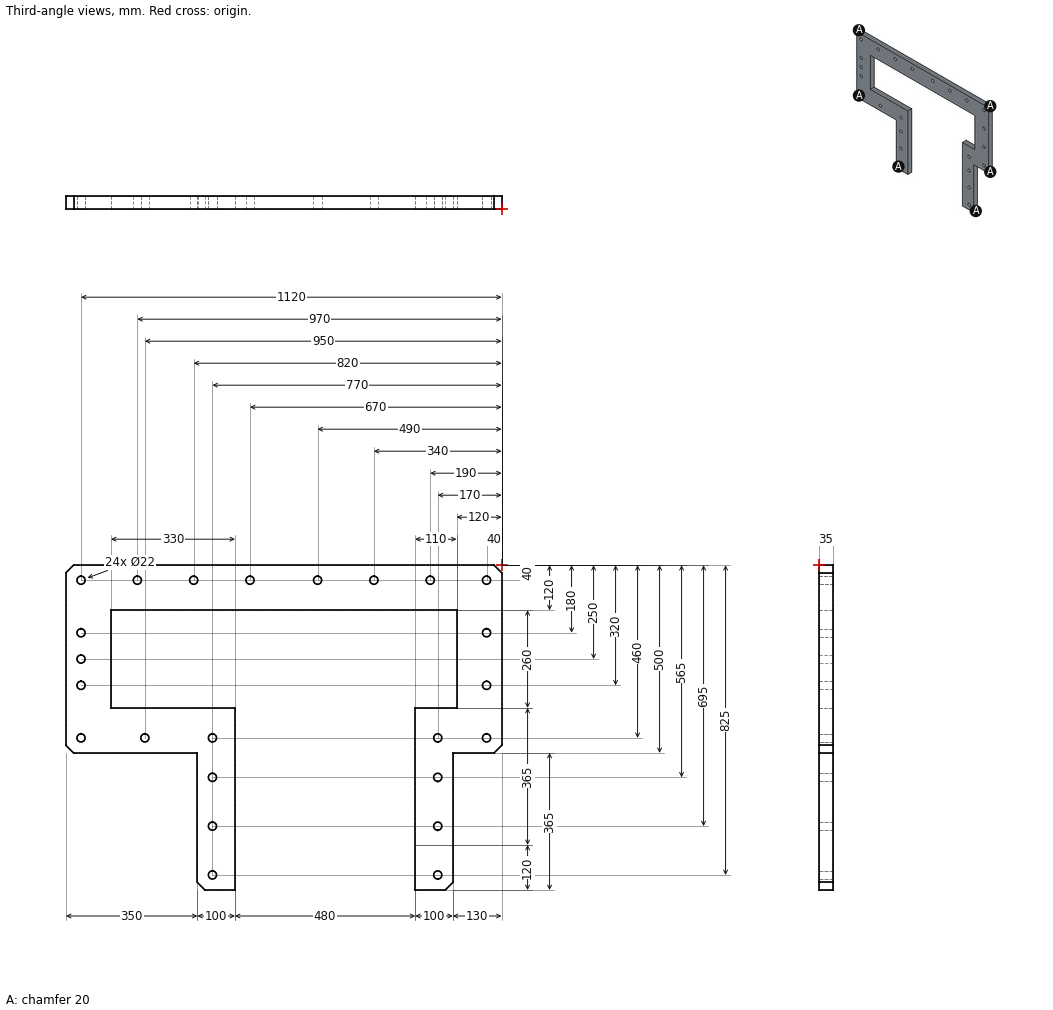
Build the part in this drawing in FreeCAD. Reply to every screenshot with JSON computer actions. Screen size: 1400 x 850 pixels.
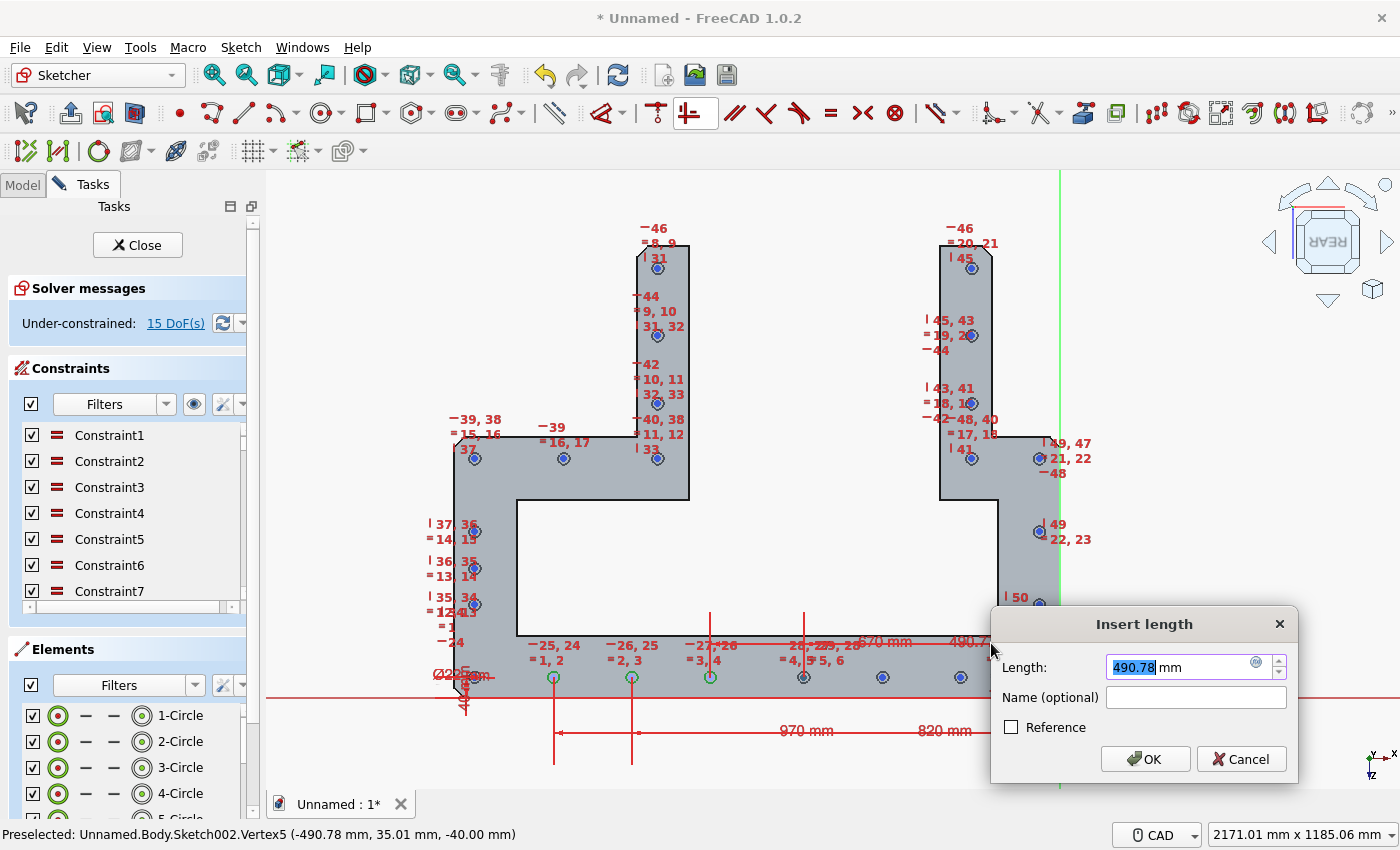
{"action": "type", "text": "490"}
{"action": "key", "text": "Return"}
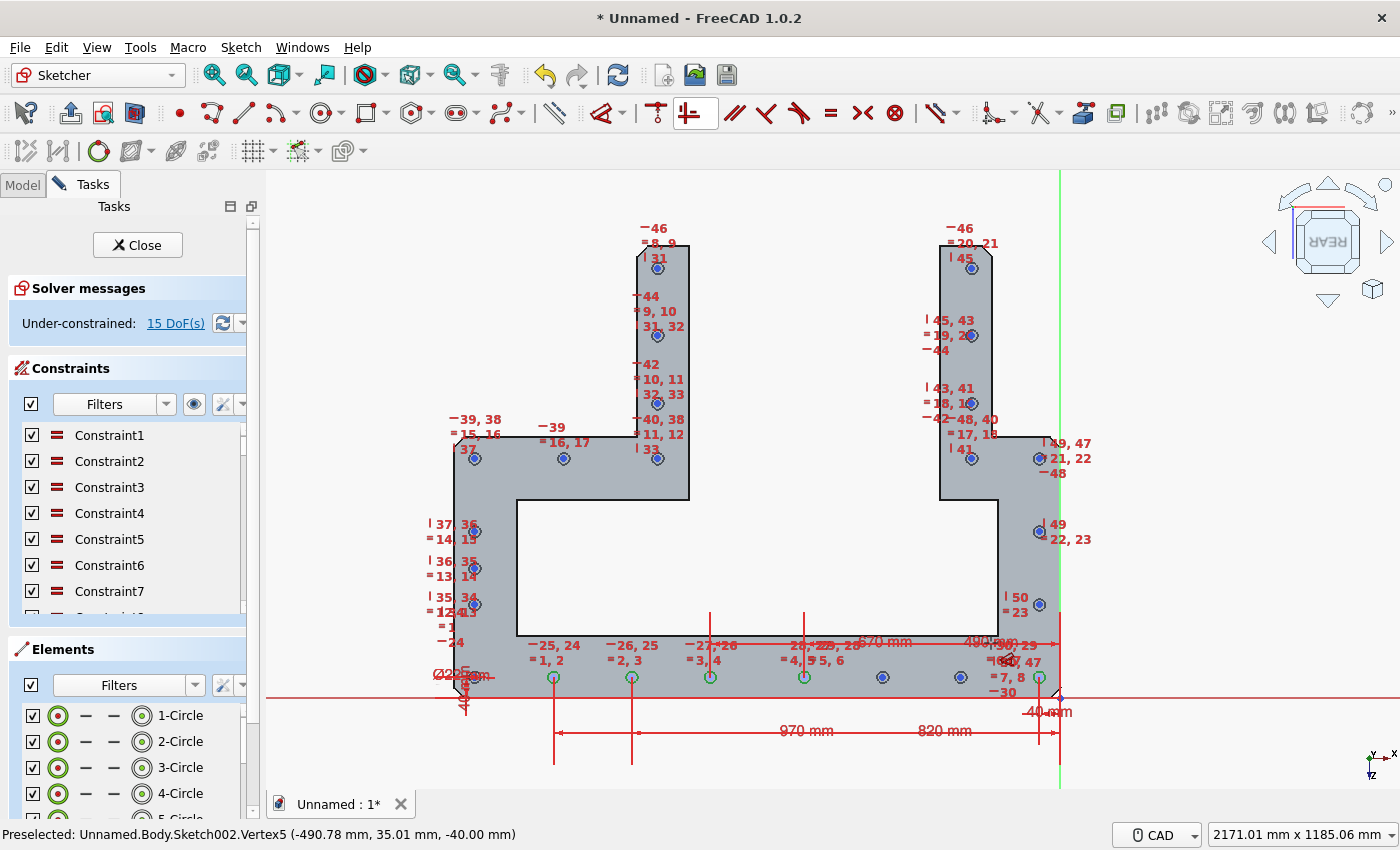
{"action": "left_click", "coordinate": [883, 677]}
{"action": "left_click", "coordinate": [972, 756]}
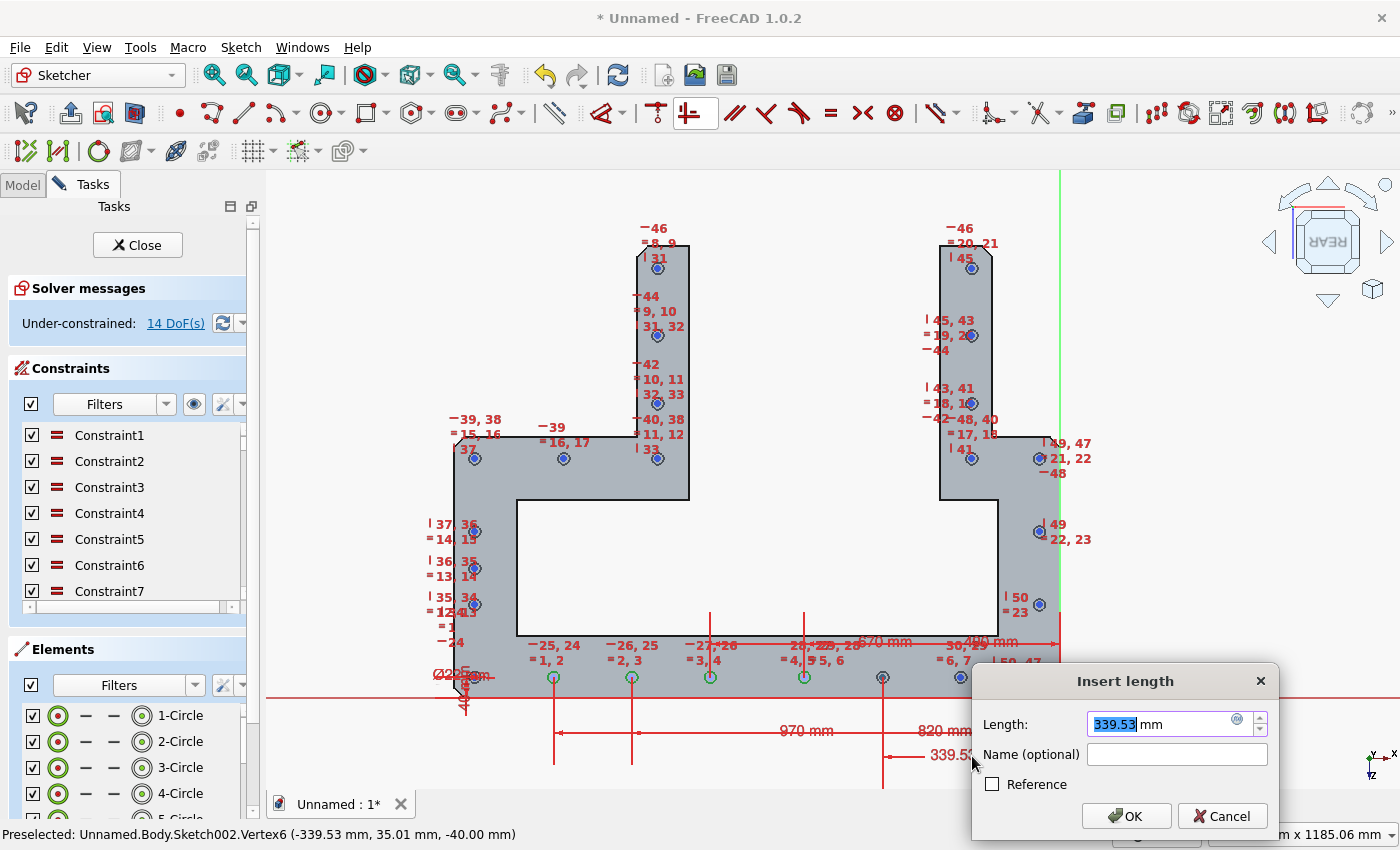
{"action": "type", "text": "340"}
{"action": "key", "text": "Return"}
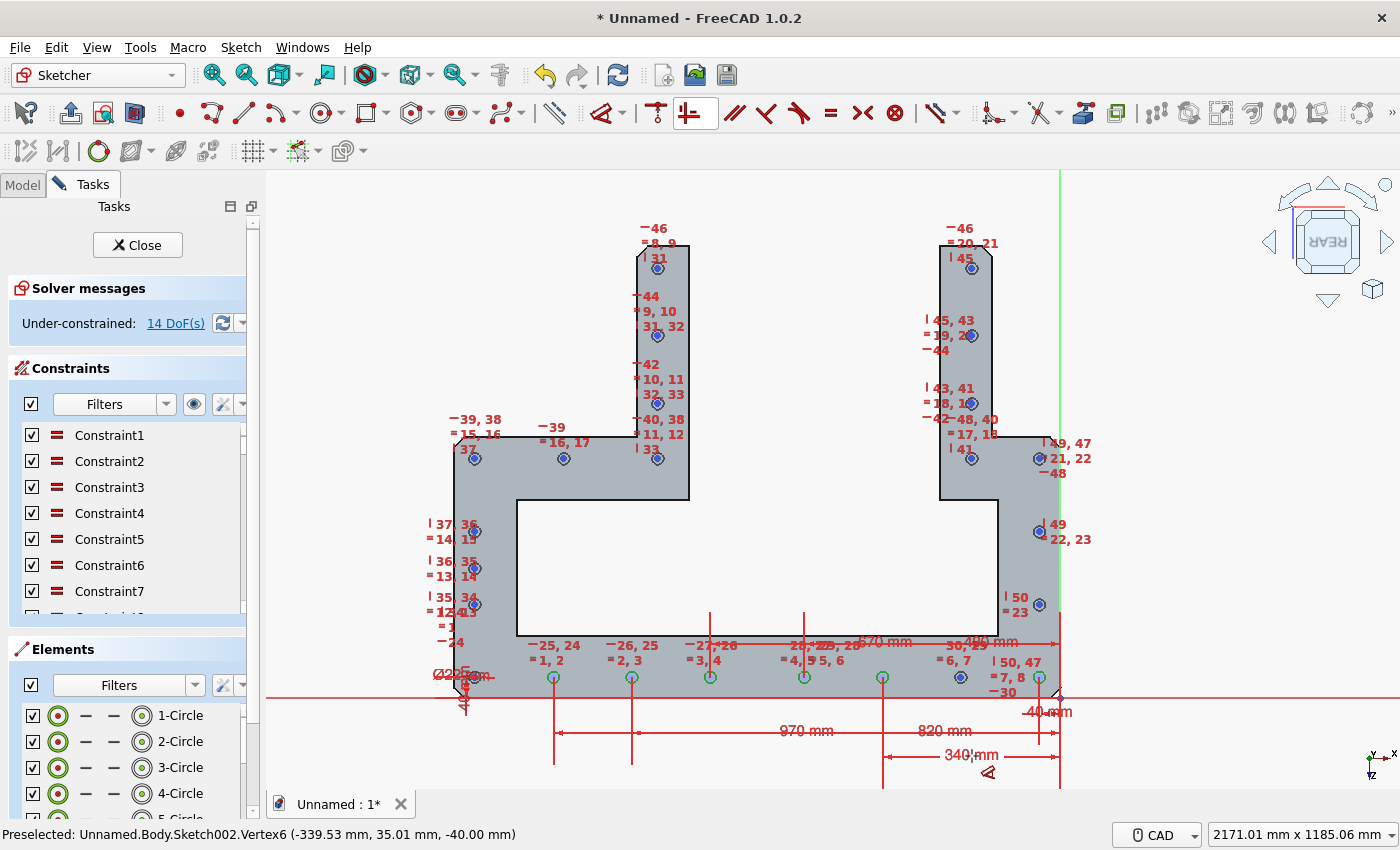
{"action": "left_click", "coordinate": [961, 677]}
{"action": "left_click", "coordinate": [1045, 756]}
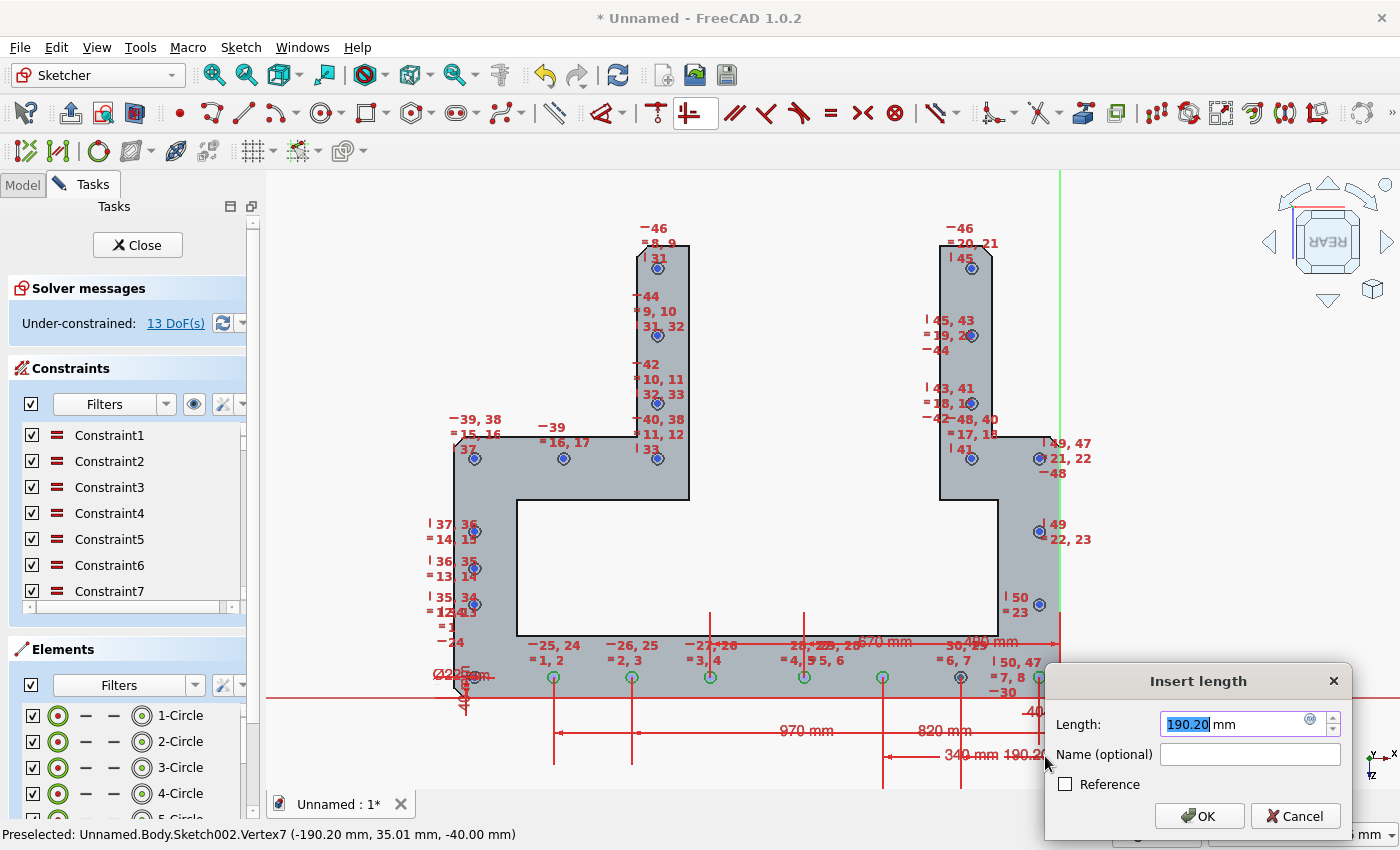
{"action": "type", "text": "190"}
{"action": "key", "text": "Return"}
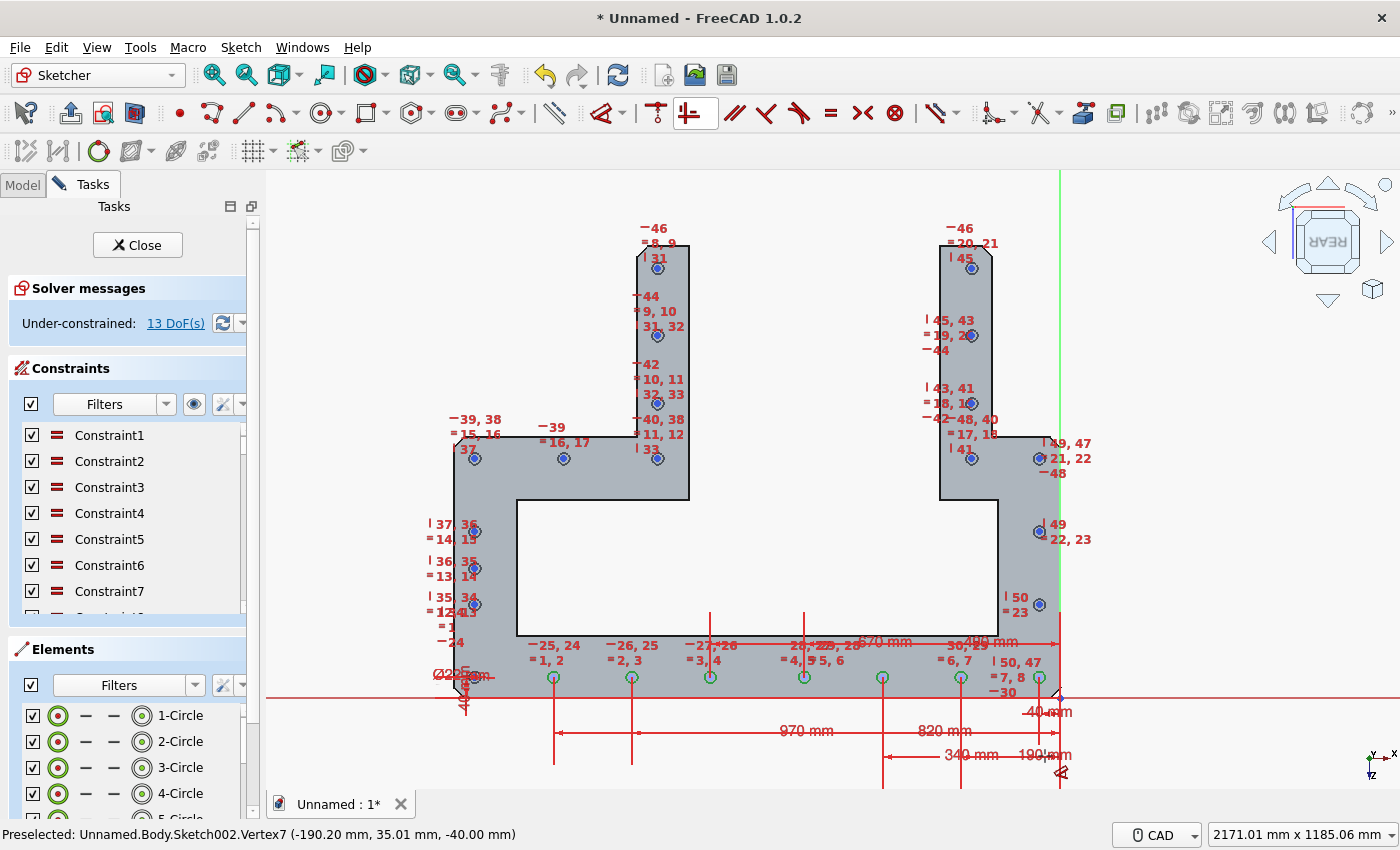
{"action": "left_click", "coordinate": [658, 269]}
{"action": "left_click", "coordinate": [718, 732]}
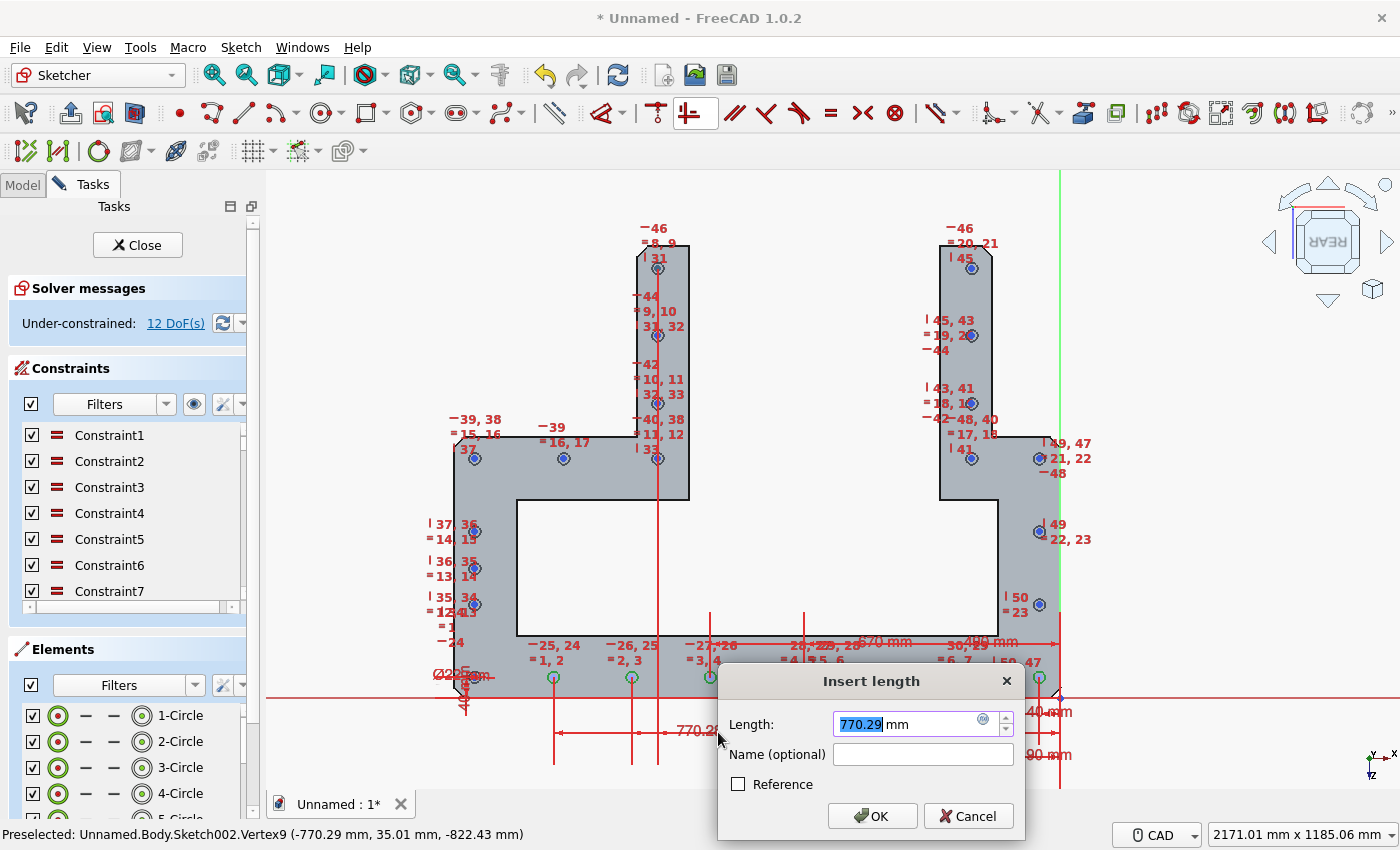
{"action": "type", "text": "770"}
{"action": "key", "text": "Return"}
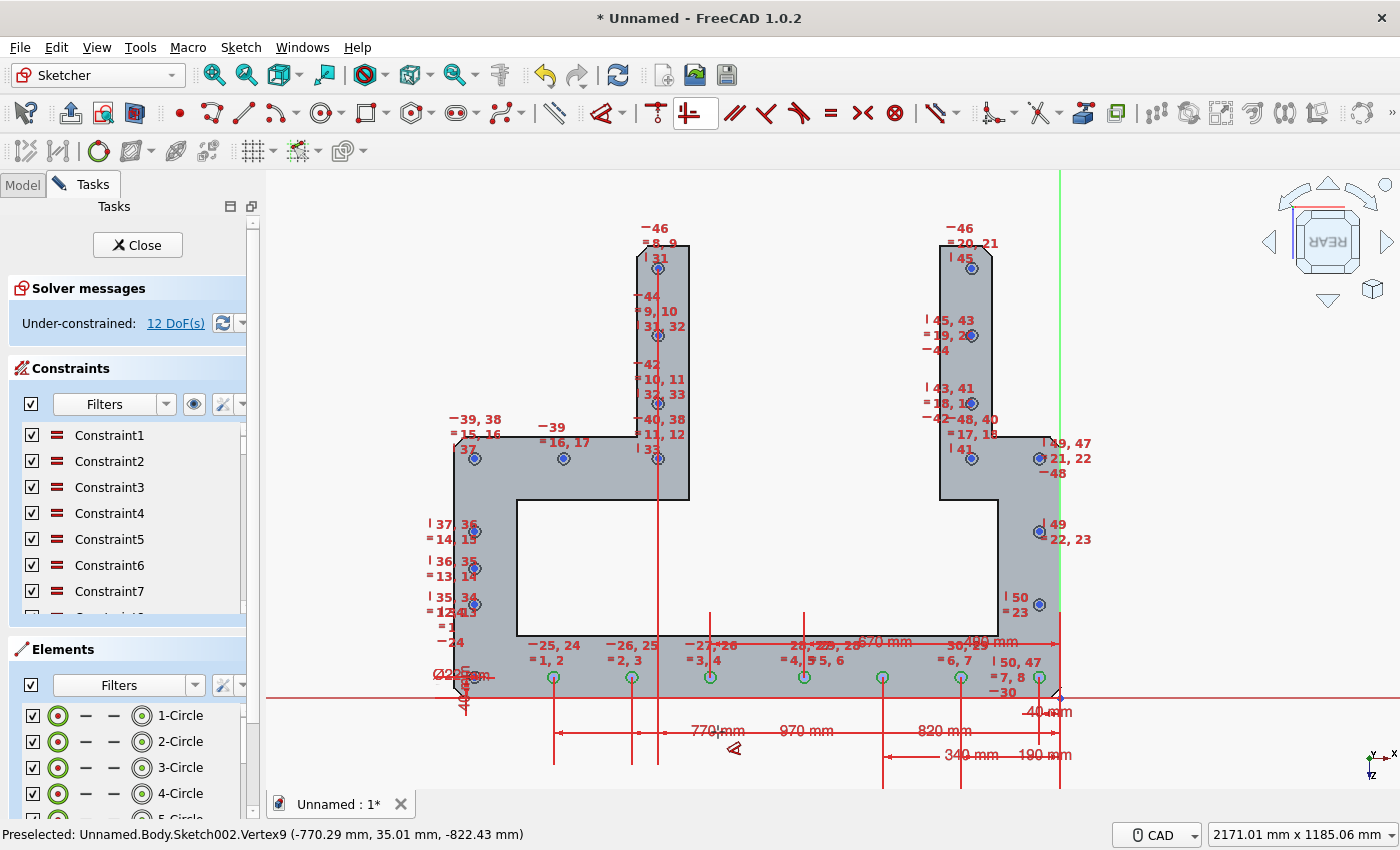
{"action": "left_click", "coordinate": [658, 269]}
{"action": "left_click", "coordinate": [1094, 483]}